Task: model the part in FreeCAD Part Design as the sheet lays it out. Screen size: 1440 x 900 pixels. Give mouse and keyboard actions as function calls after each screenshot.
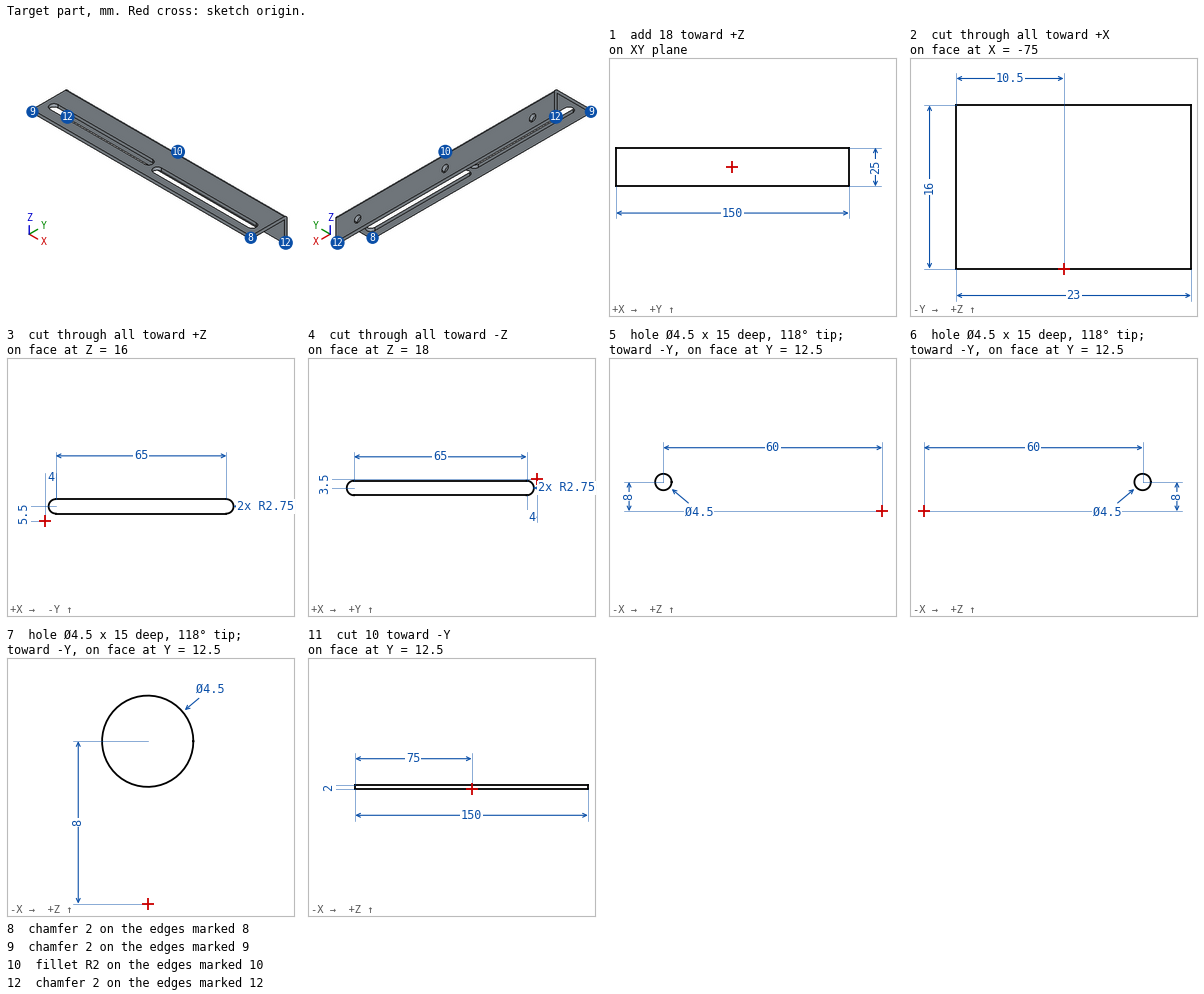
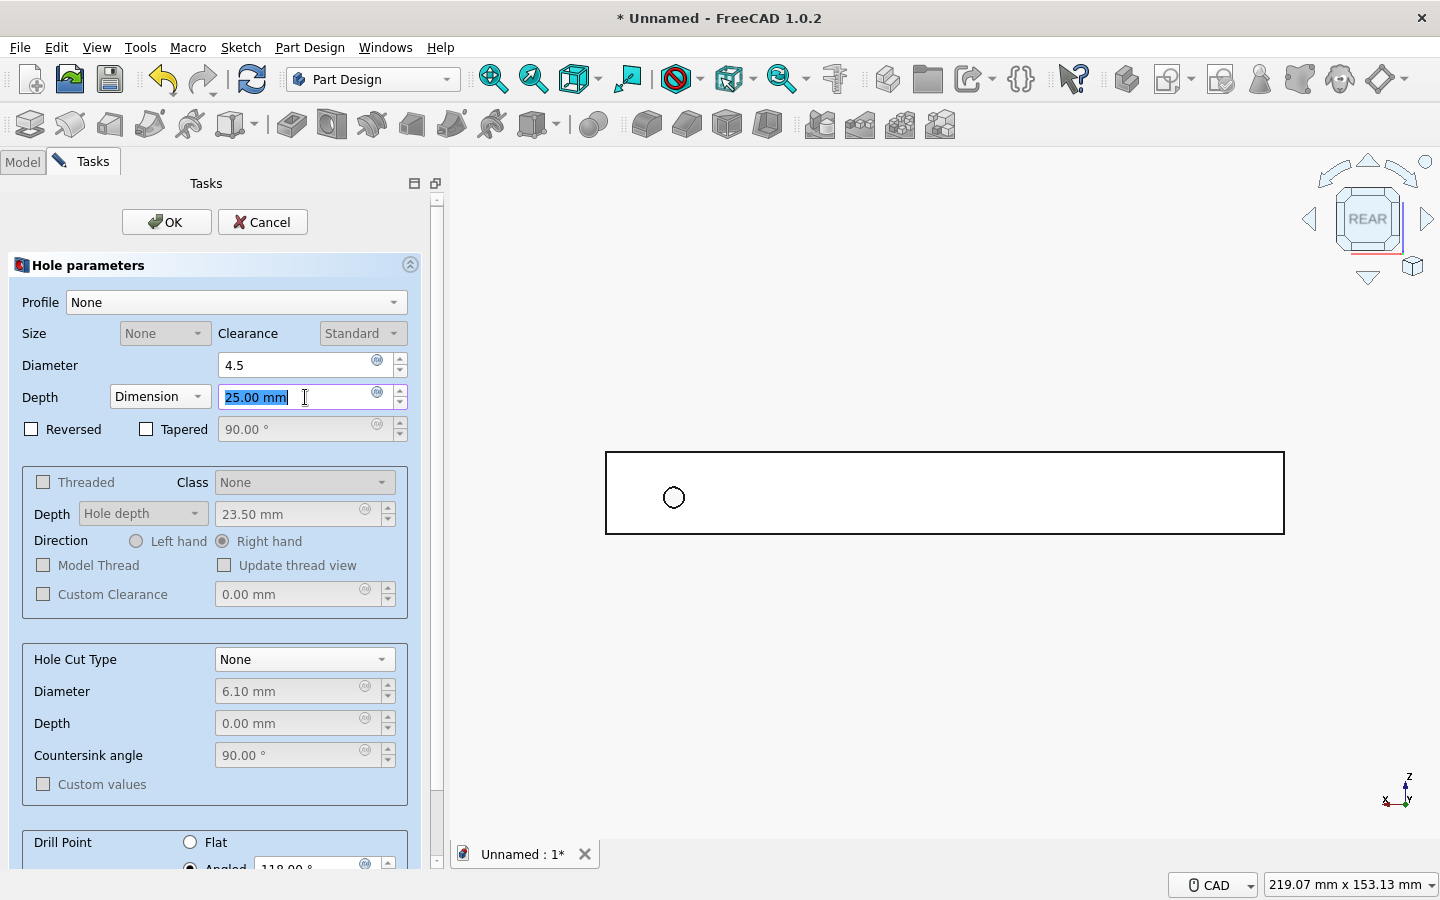
text(15)
key(Tab)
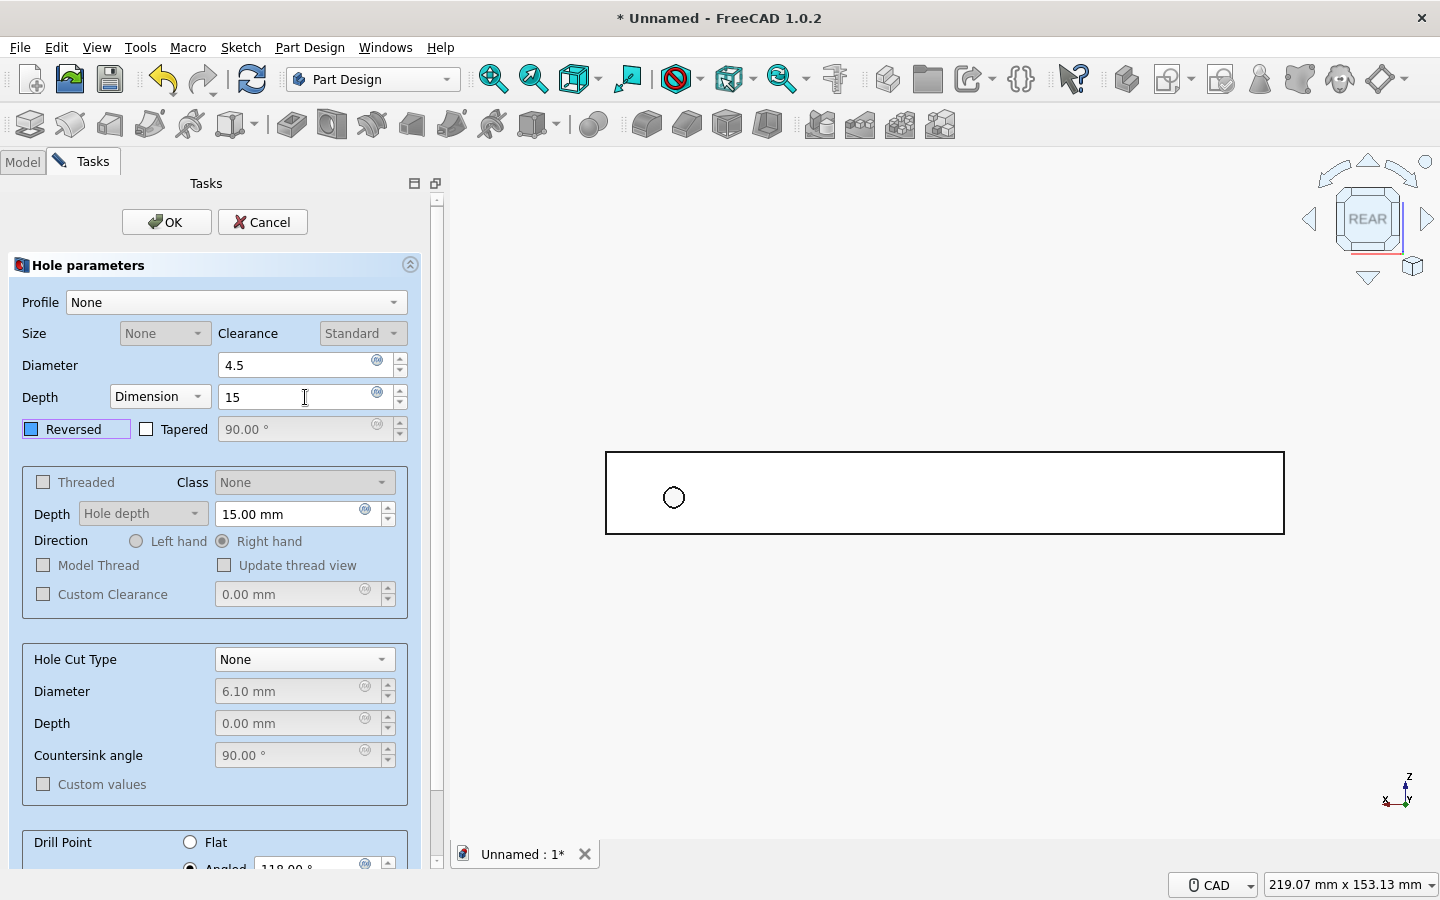
click(167, 222)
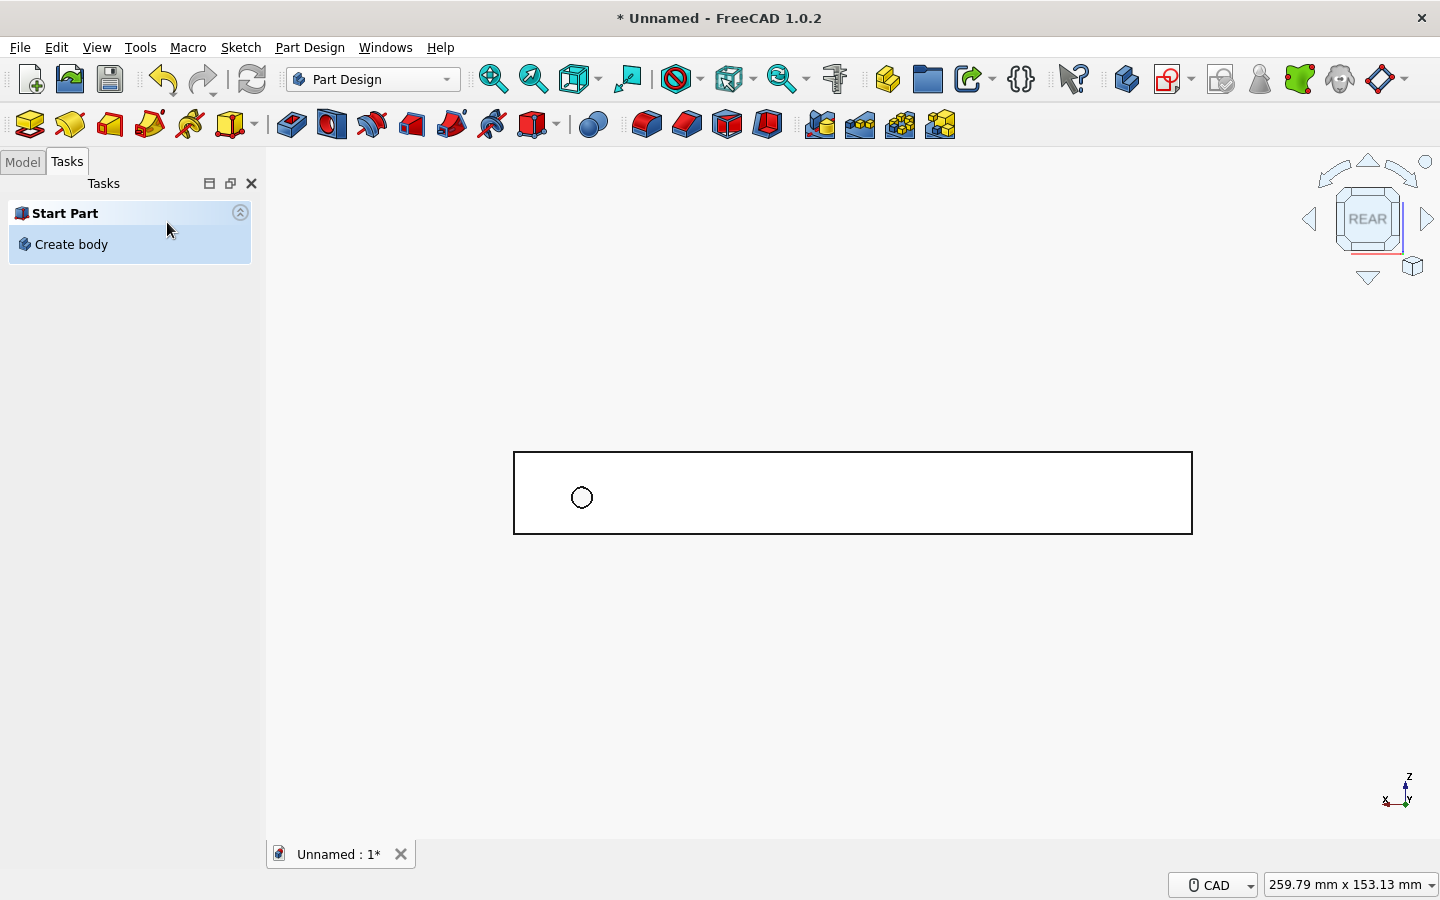
click(659, 492)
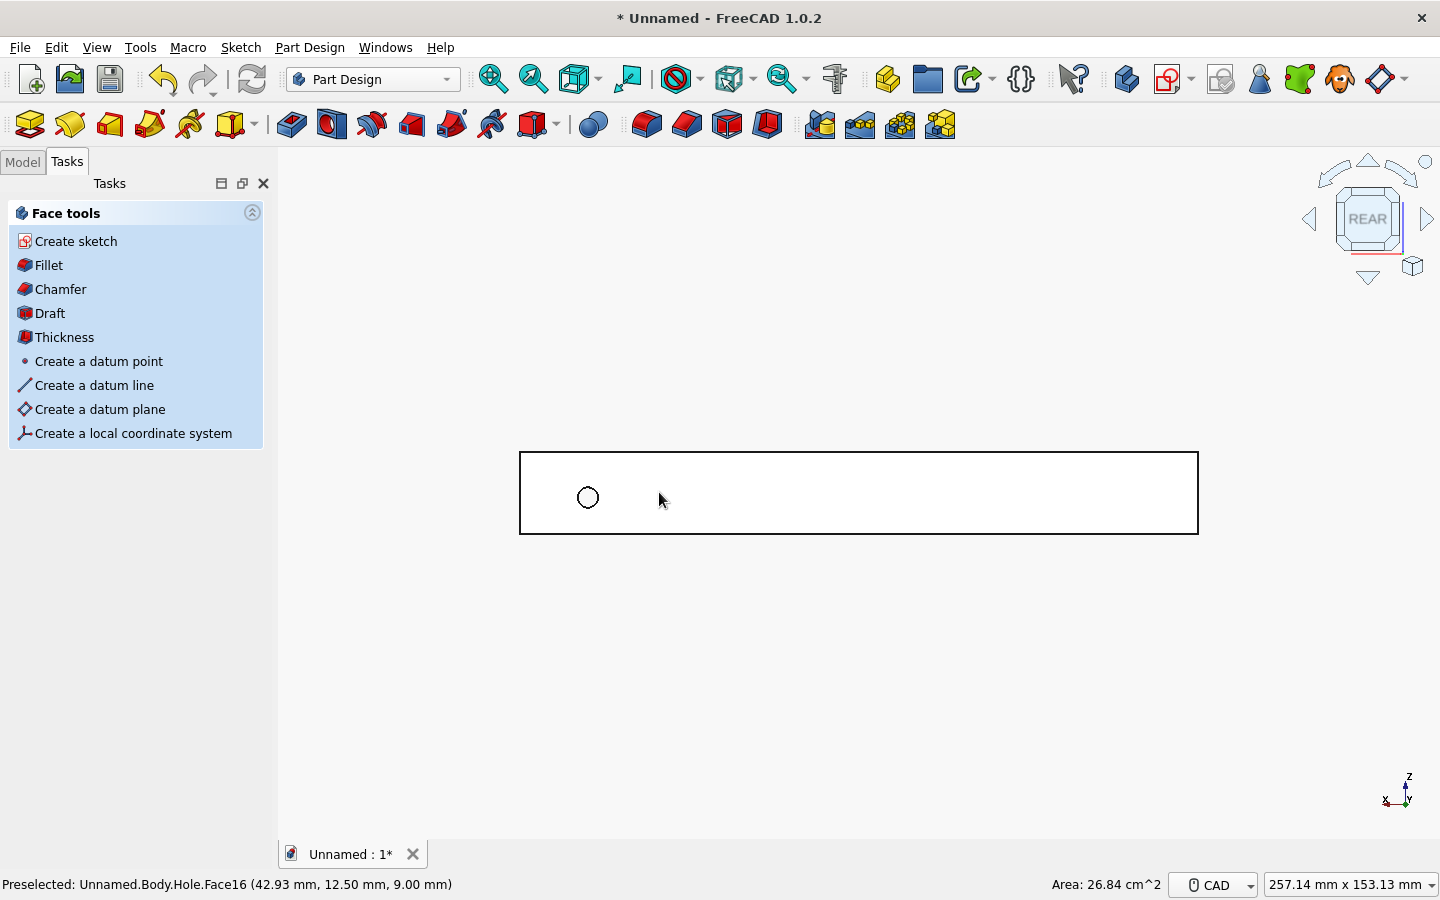
click(1168, 80)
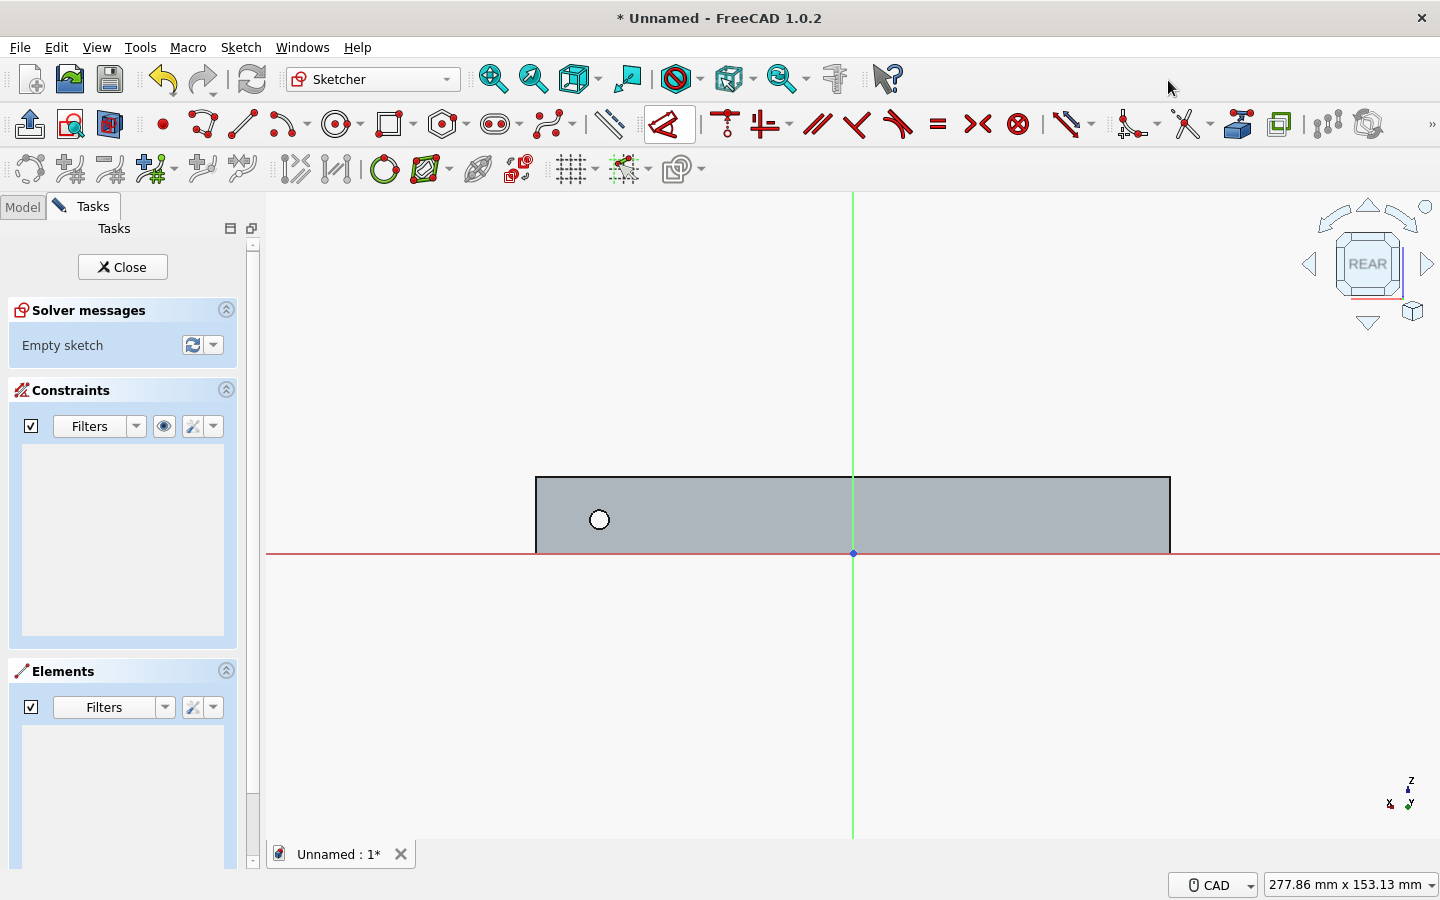
scroll(1123, 520, up, 15)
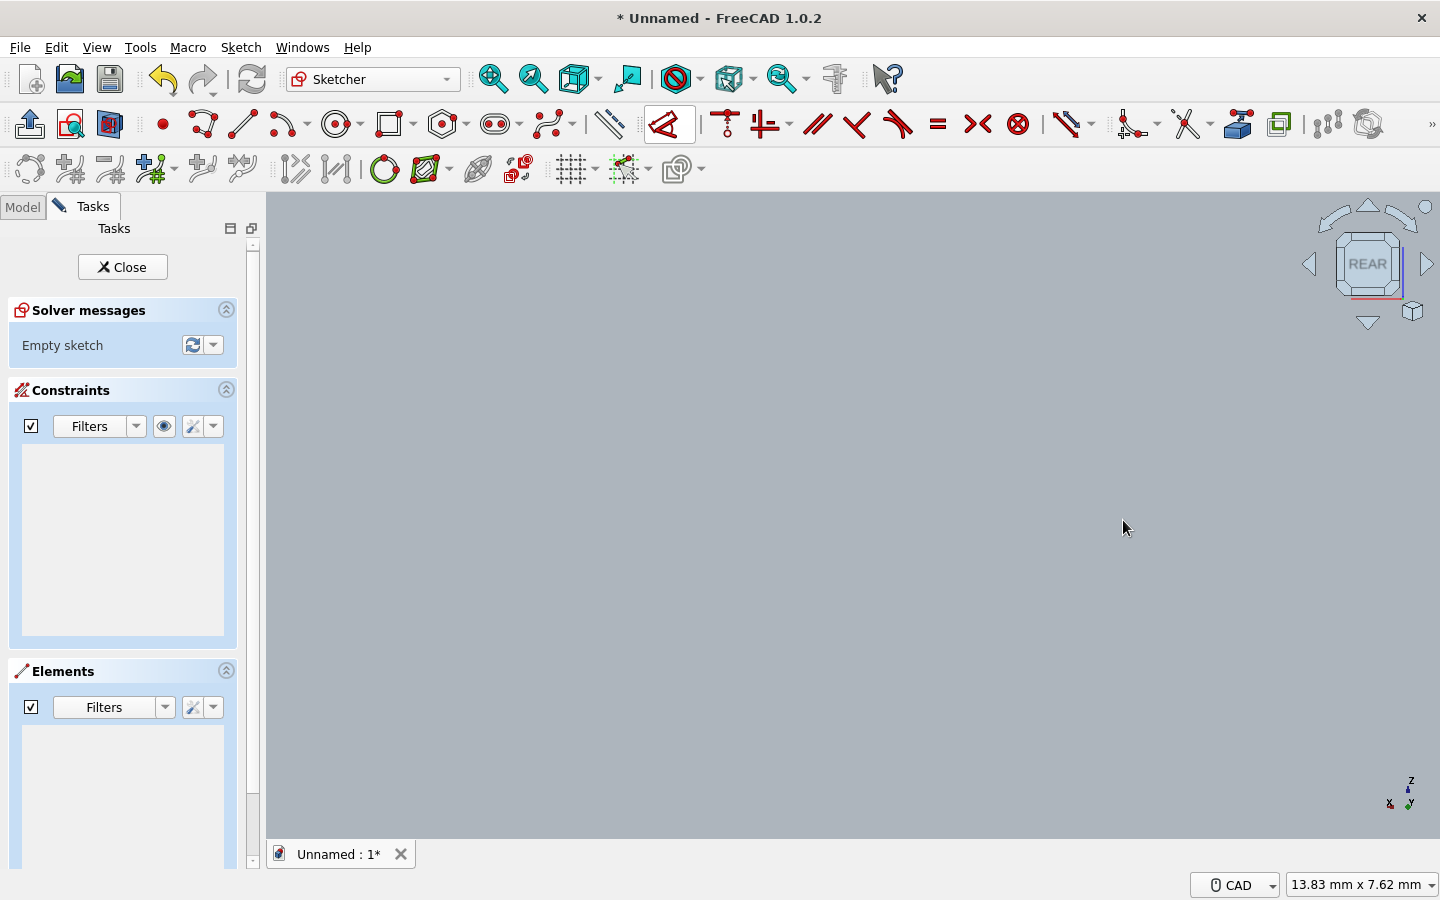
click(336, 124)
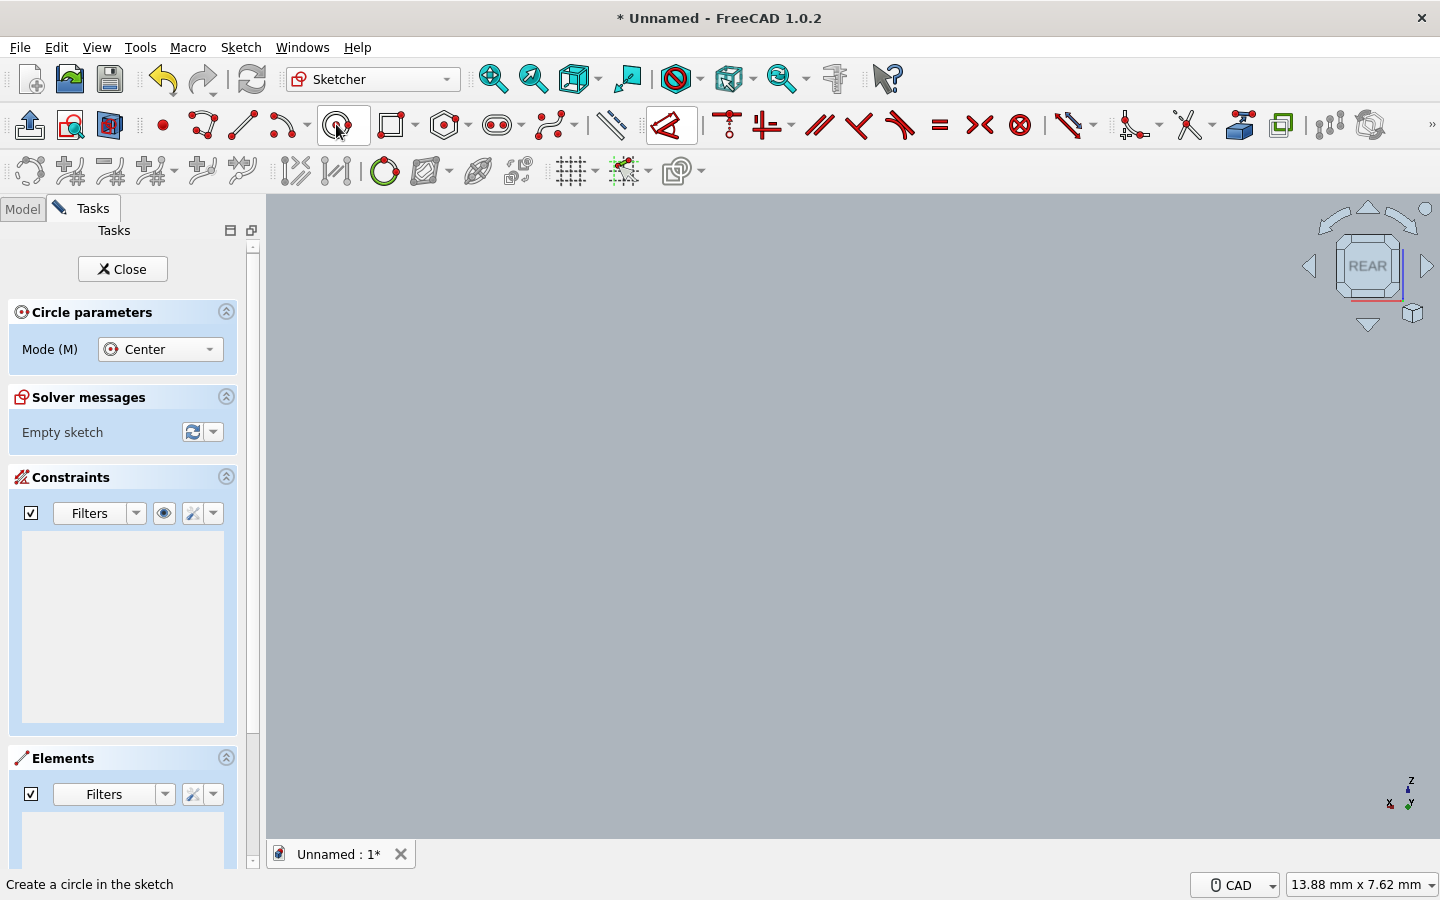
click(778, 506)
move(913, 371)